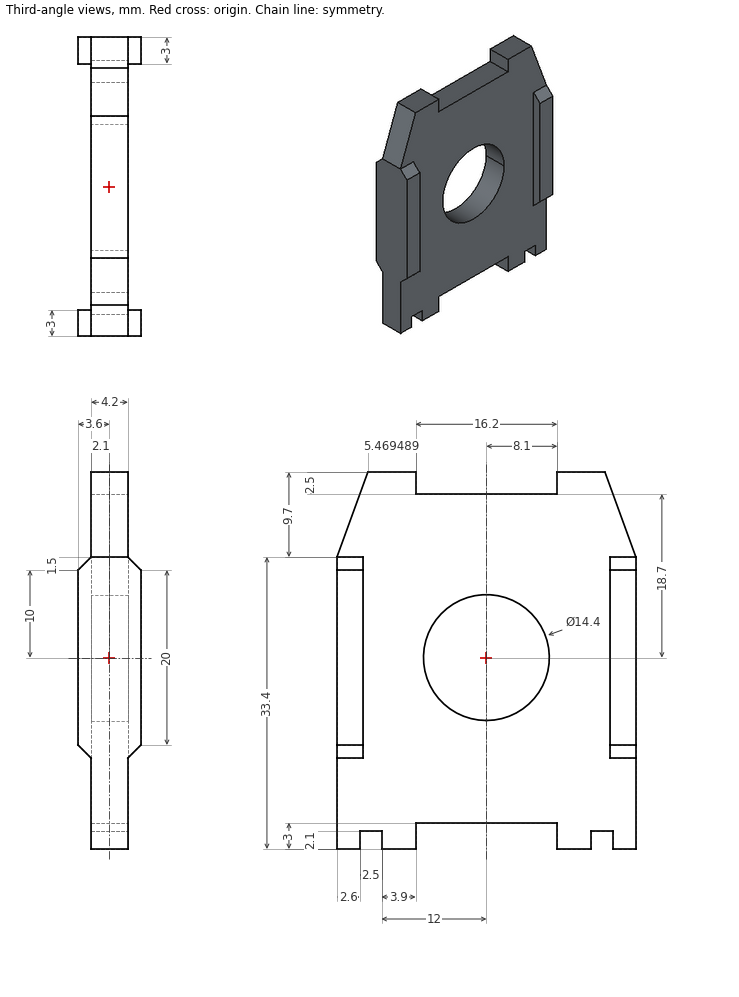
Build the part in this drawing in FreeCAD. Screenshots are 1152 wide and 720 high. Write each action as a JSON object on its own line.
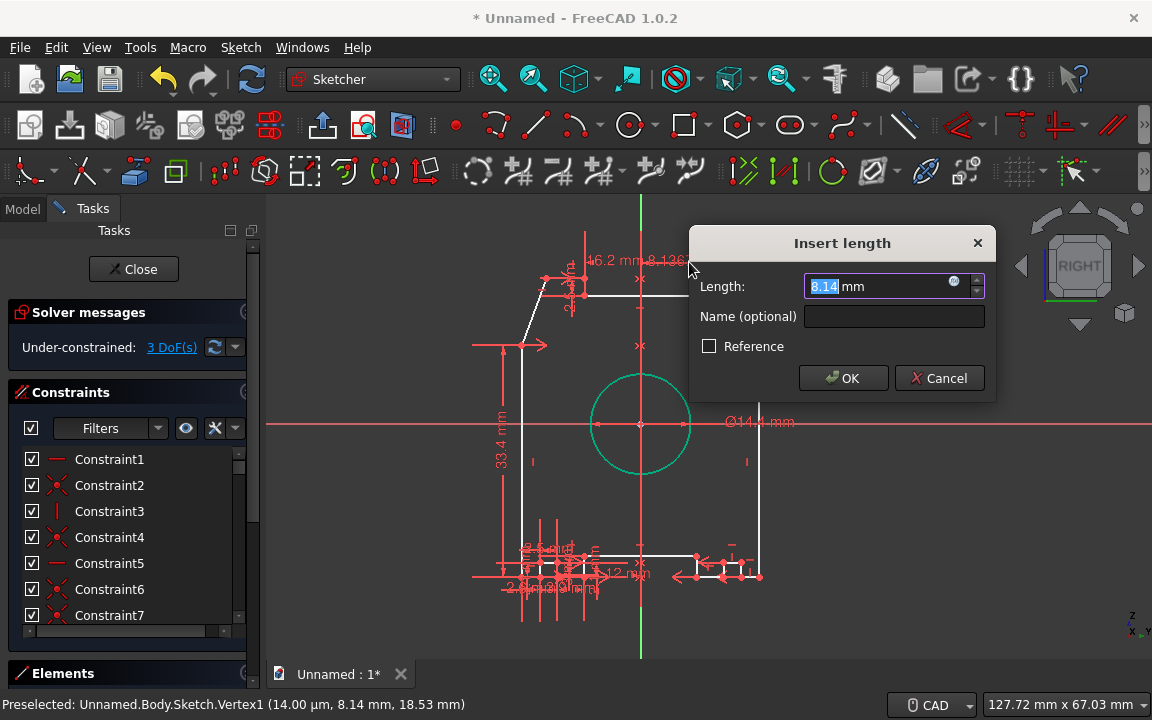
{"action": "type", "text": "8.1"}
{"action": "key", "text": "Return"}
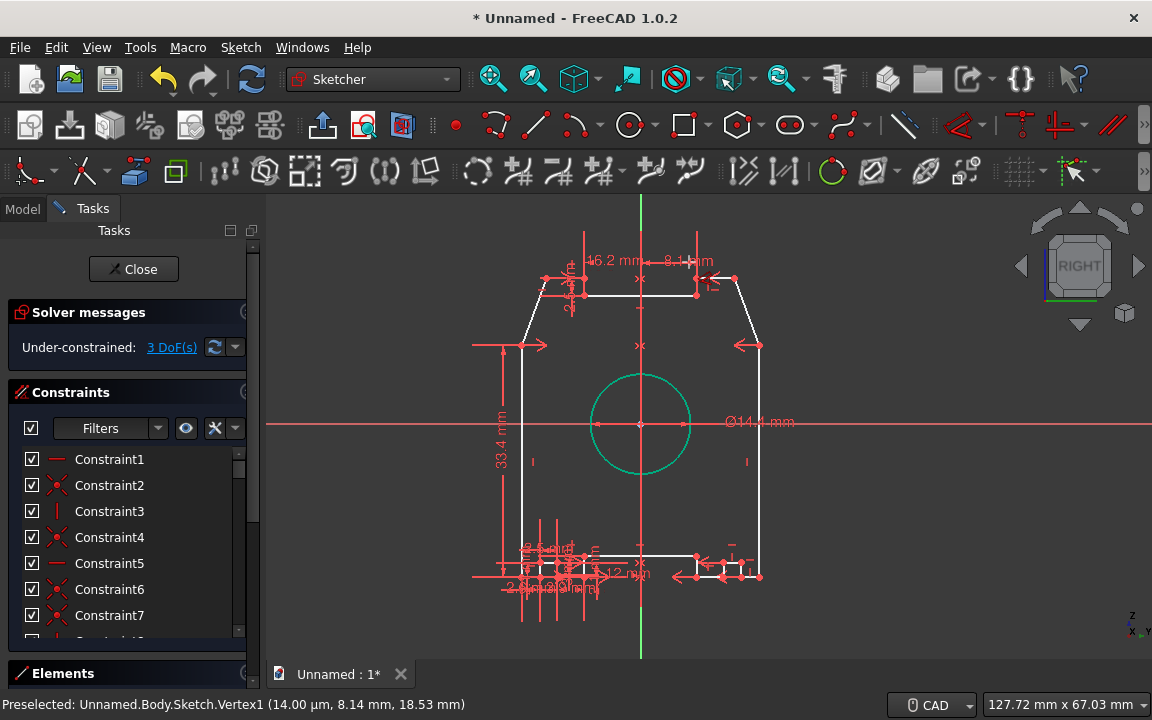
{"action": "left_click", "coordinate": [539, 298]}
{"action": "left_click", "coordinate": [488, 312]}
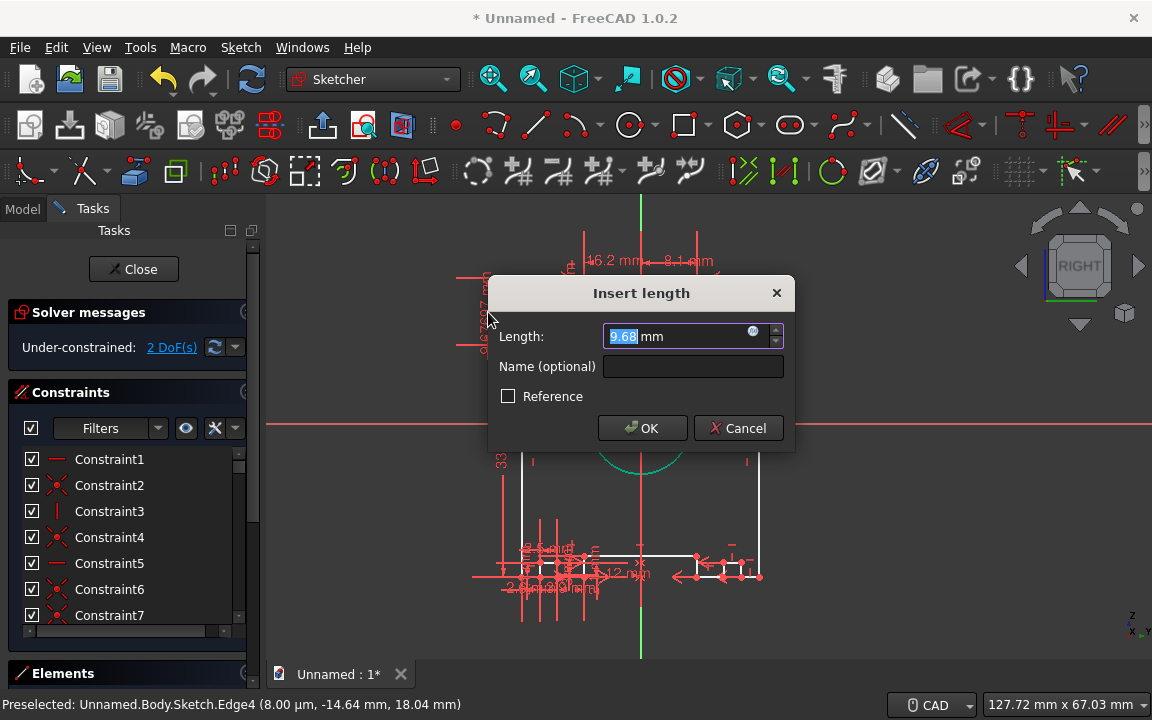
{"action": "type", "text": "9.7"}
{"action": "key", "text": "Return"}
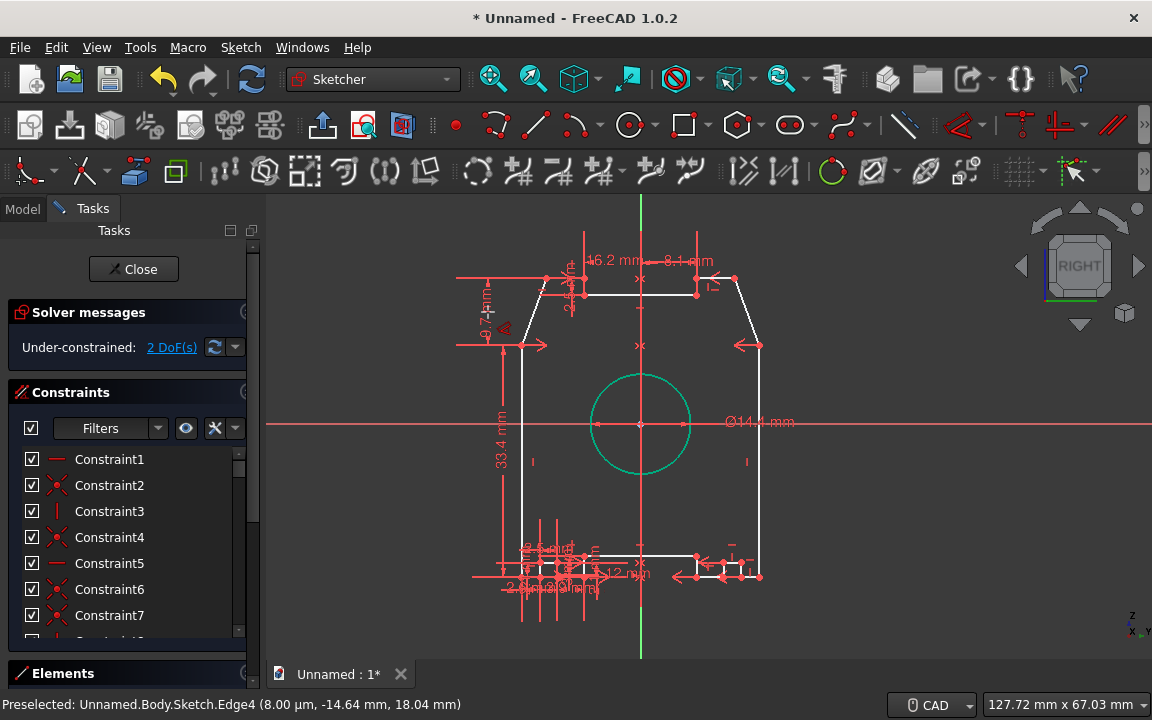
{"action": "left_click", "coordinate": [697, 295]}
{"action": "left_click", "coordinate": [731, 360]}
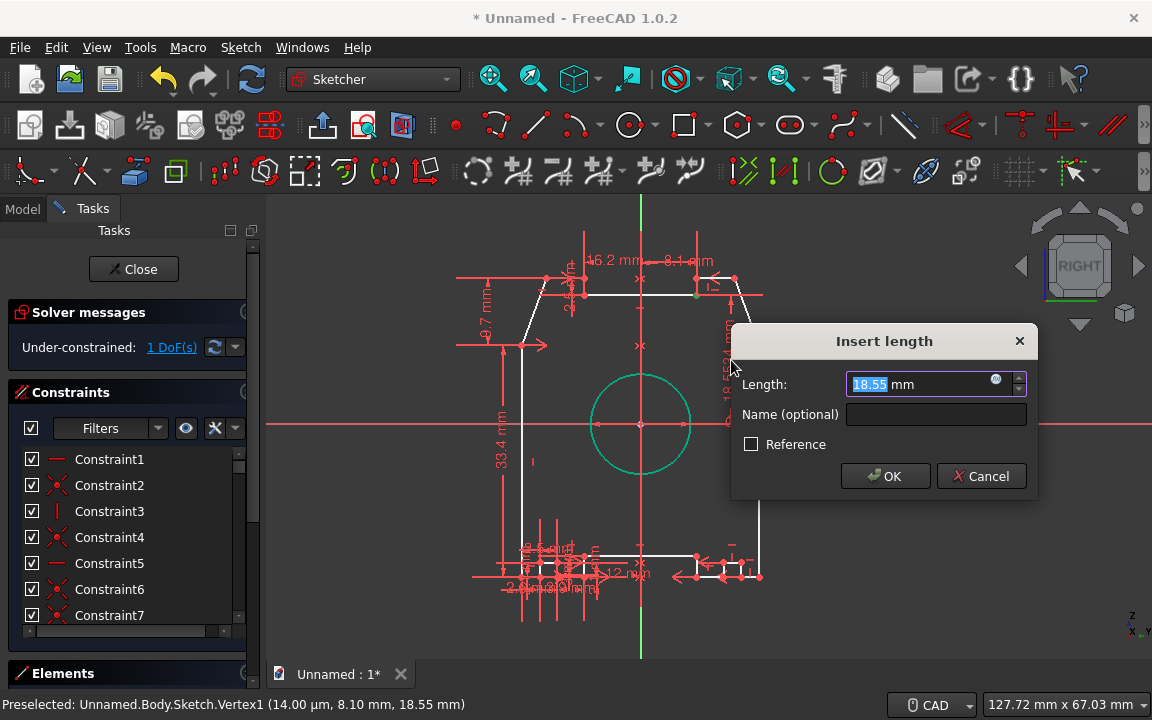
{"action": "type", "text": "18.7"}
{"action": "key", "text": "Return"}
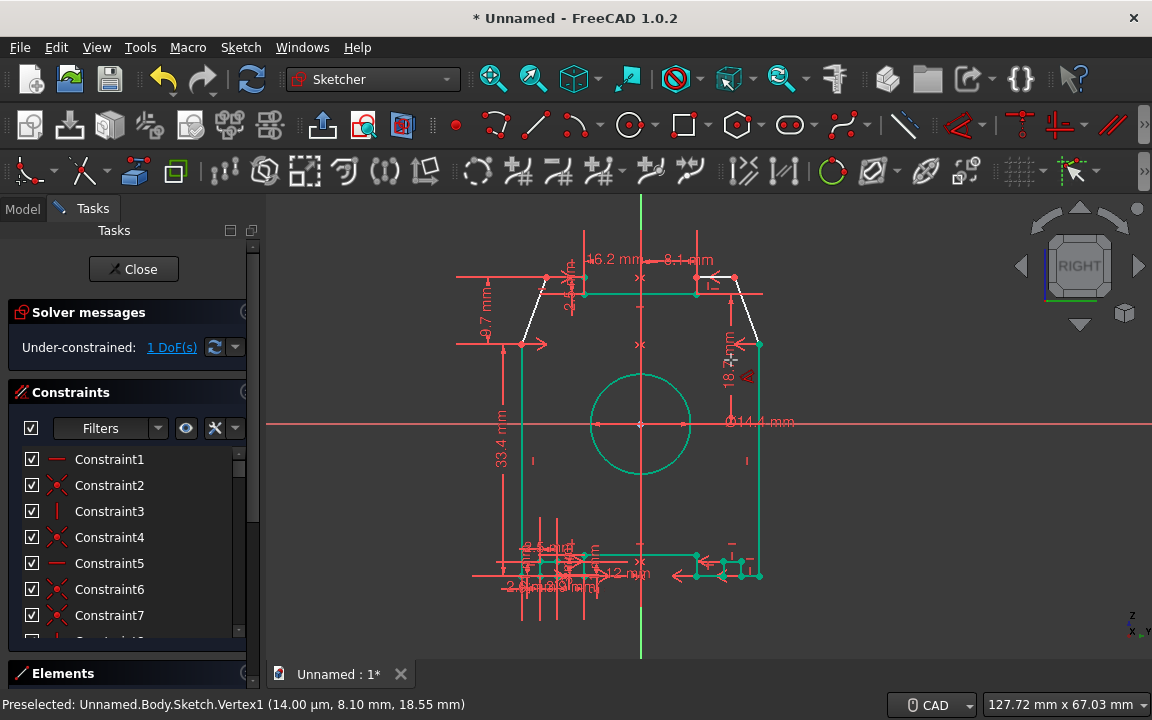
{"action": "left_click", "coordinate": [573, 277]}
{"action": "left_click", "coordinate": [566, 311]}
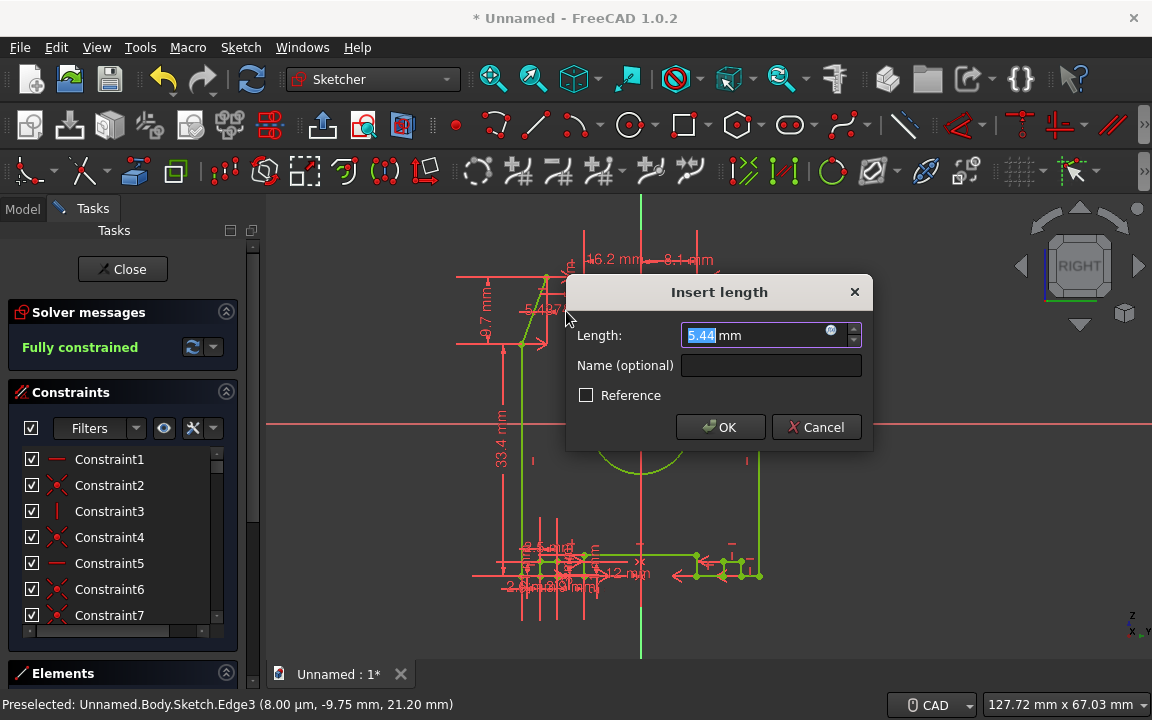
{"action": "type", "text": "5.469489"}
{"action": "key", "text": "Return"}
{"action": "key", "text": "Escape"}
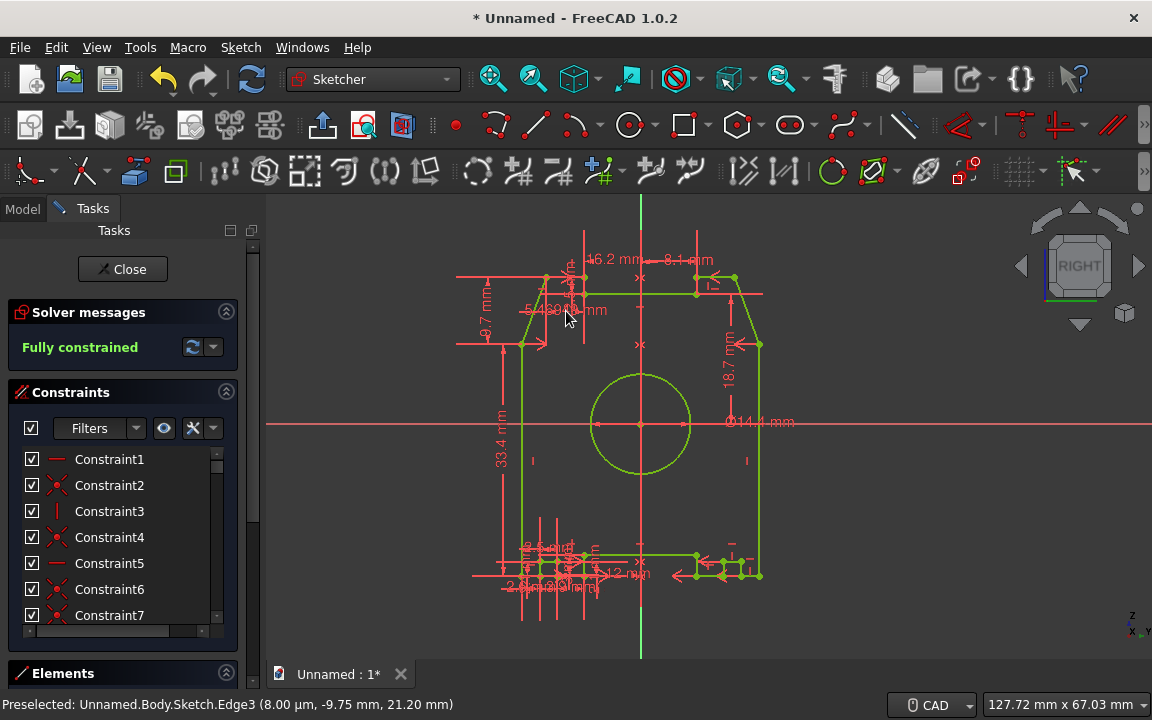
{"action": "left_click", "coordinate": [123, 269]}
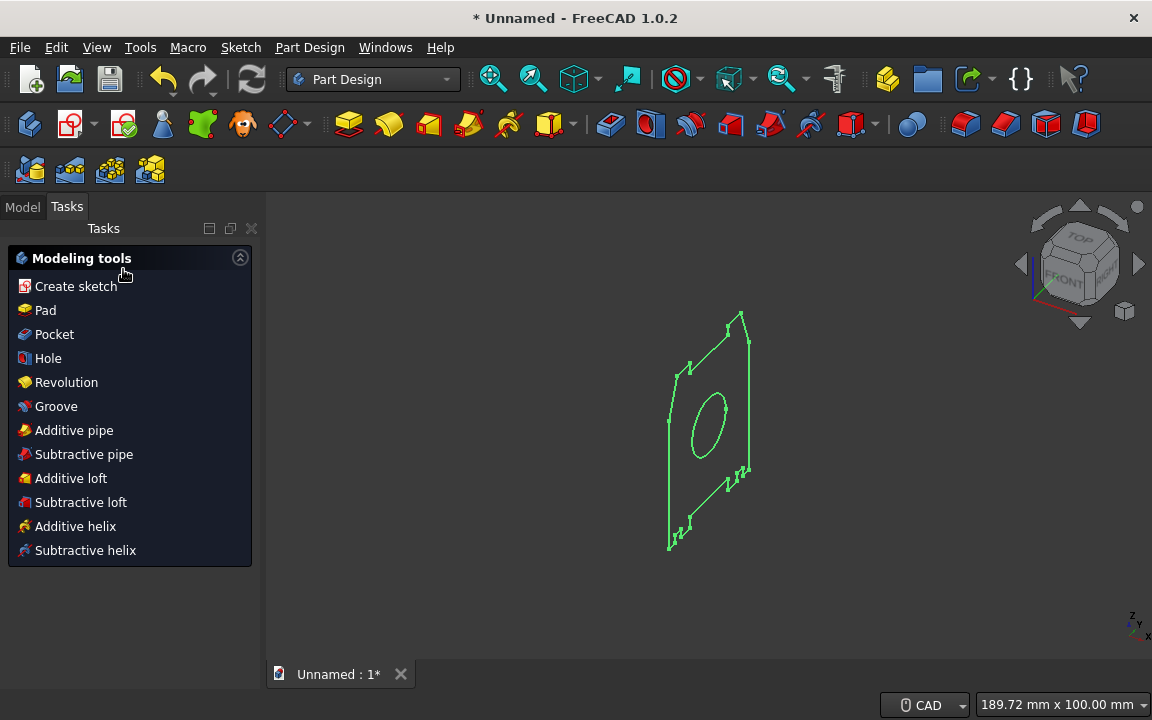
{"action": "left_click", "coordinate": [350, 124]}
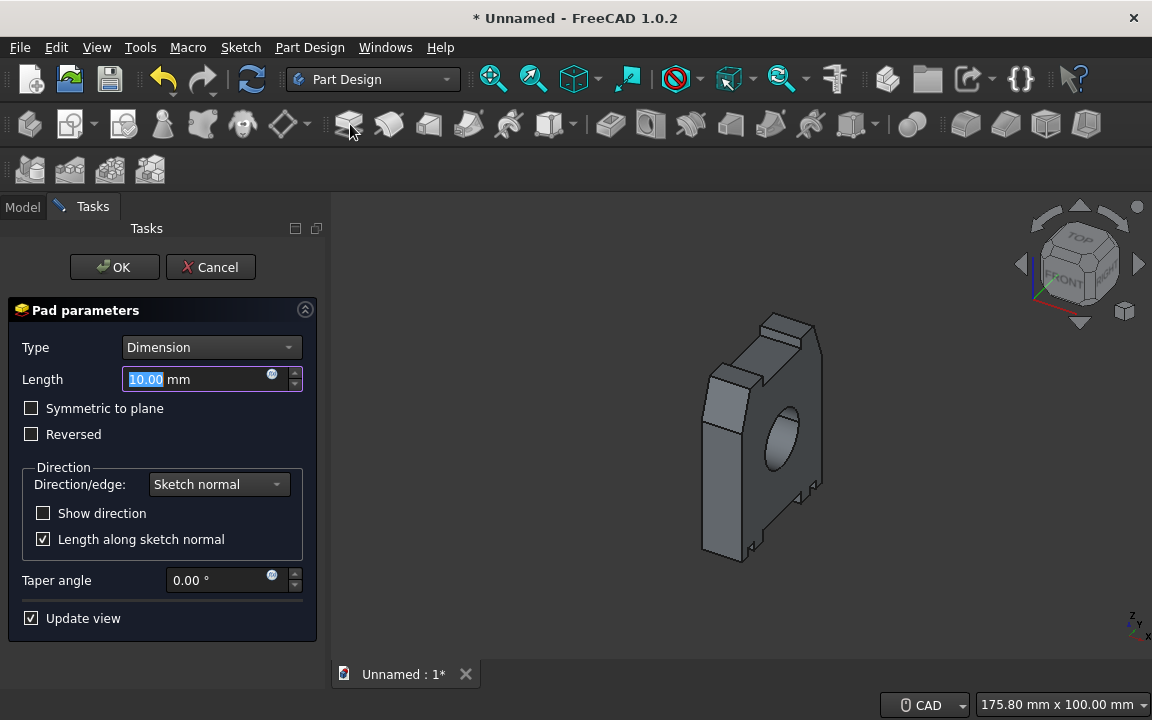
{"action": "type", "text": "4.2"}
{"action": "key", "text": "Tab"}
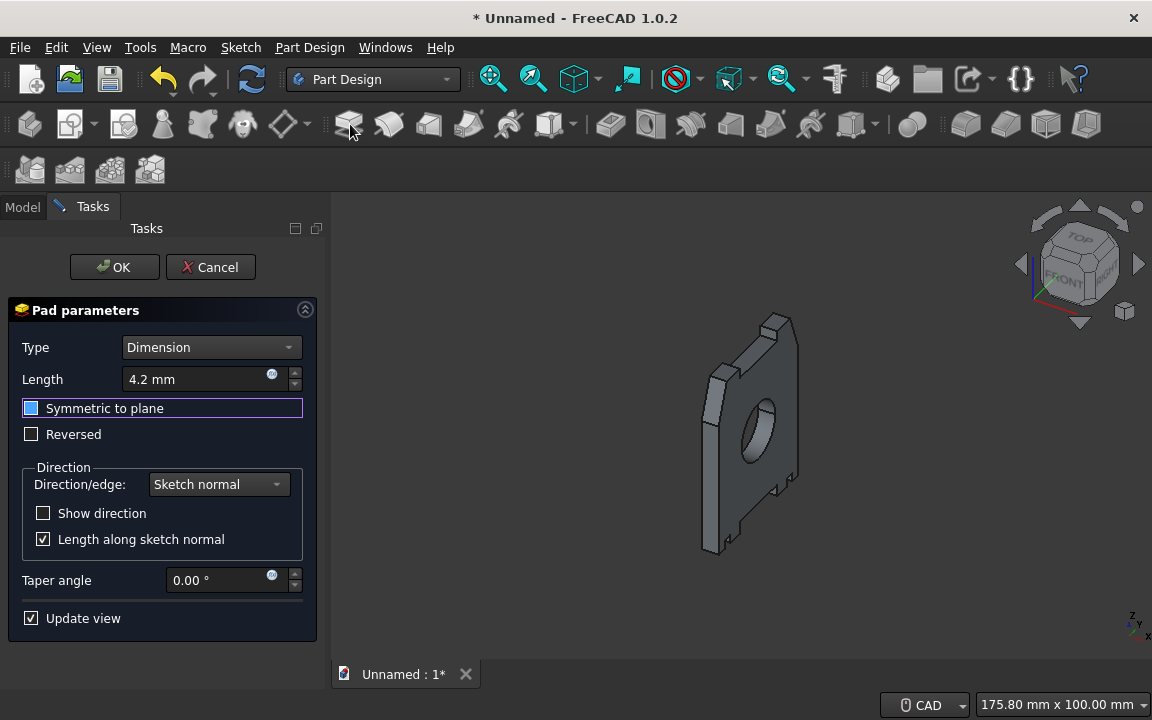
{"action": "left_click", "coordinate": [30, 408]}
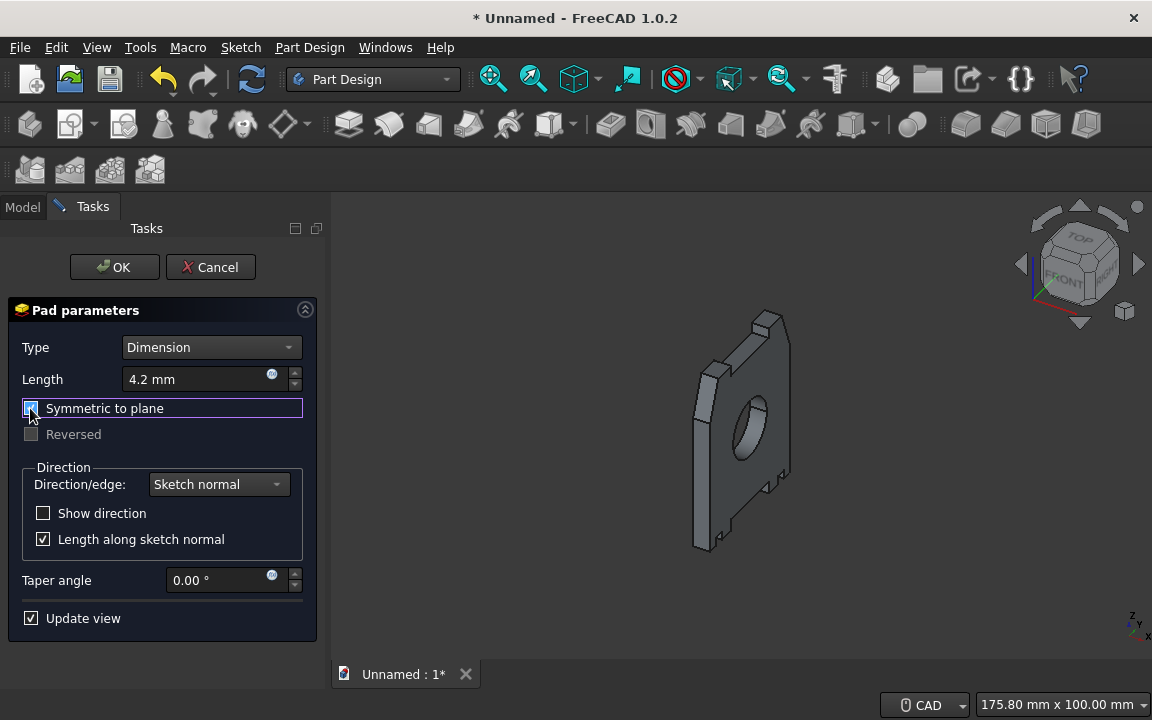
{"action": "left_click", "coordinate": [115, 267]}